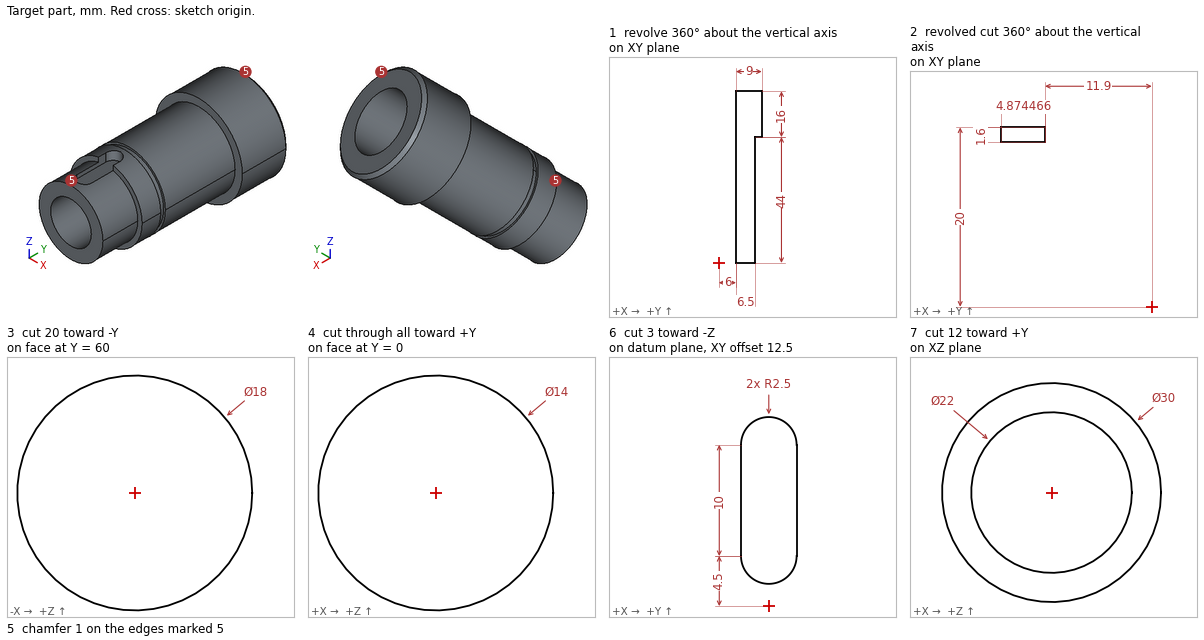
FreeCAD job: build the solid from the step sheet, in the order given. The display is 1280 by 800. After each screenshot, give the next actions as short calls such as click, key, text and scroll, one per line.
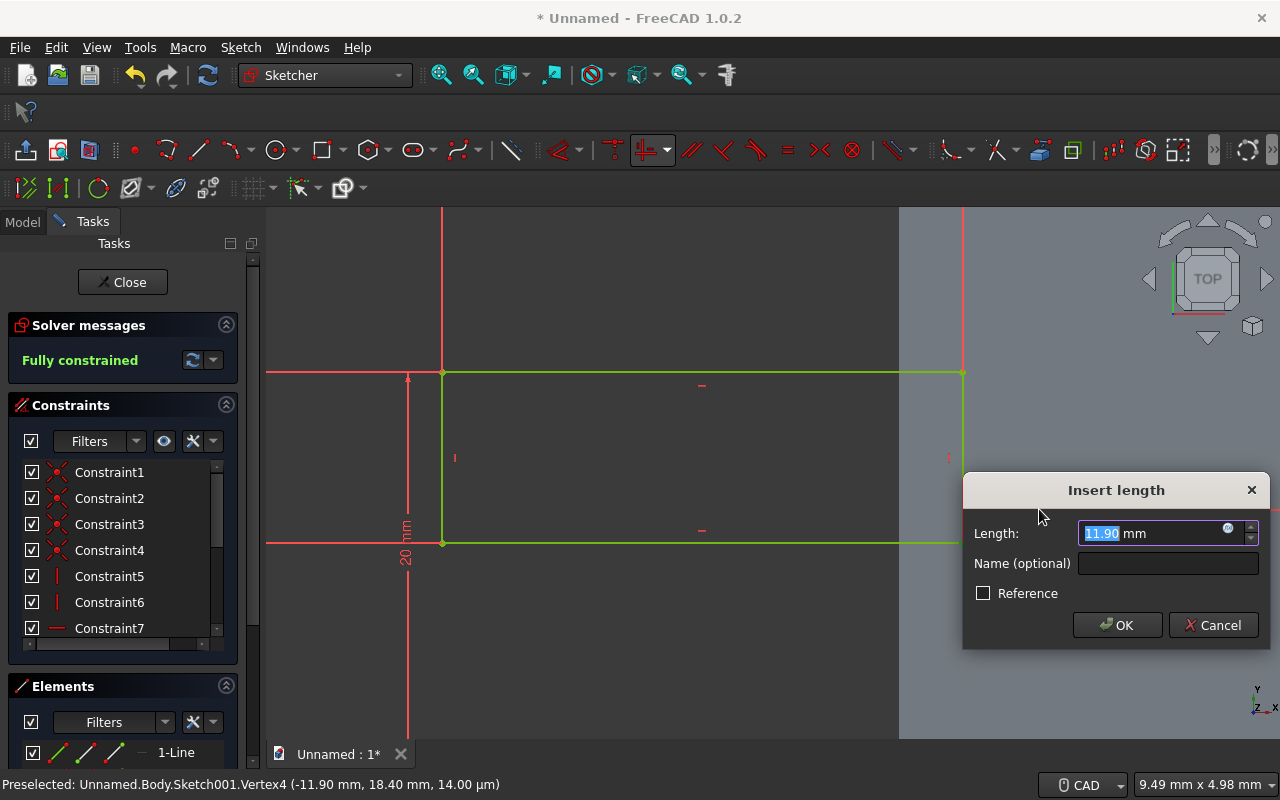
text(11.9)
key(Return)
key(Escape)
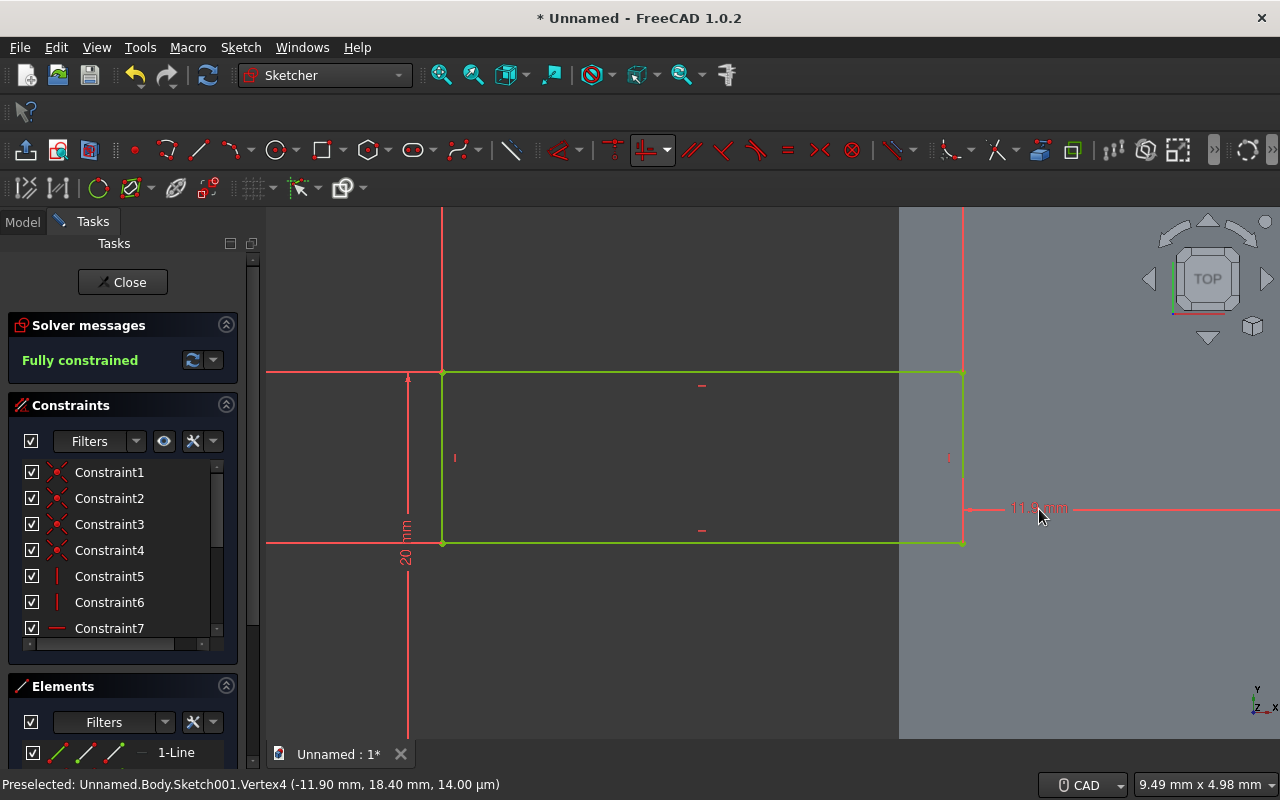
click(123, 282)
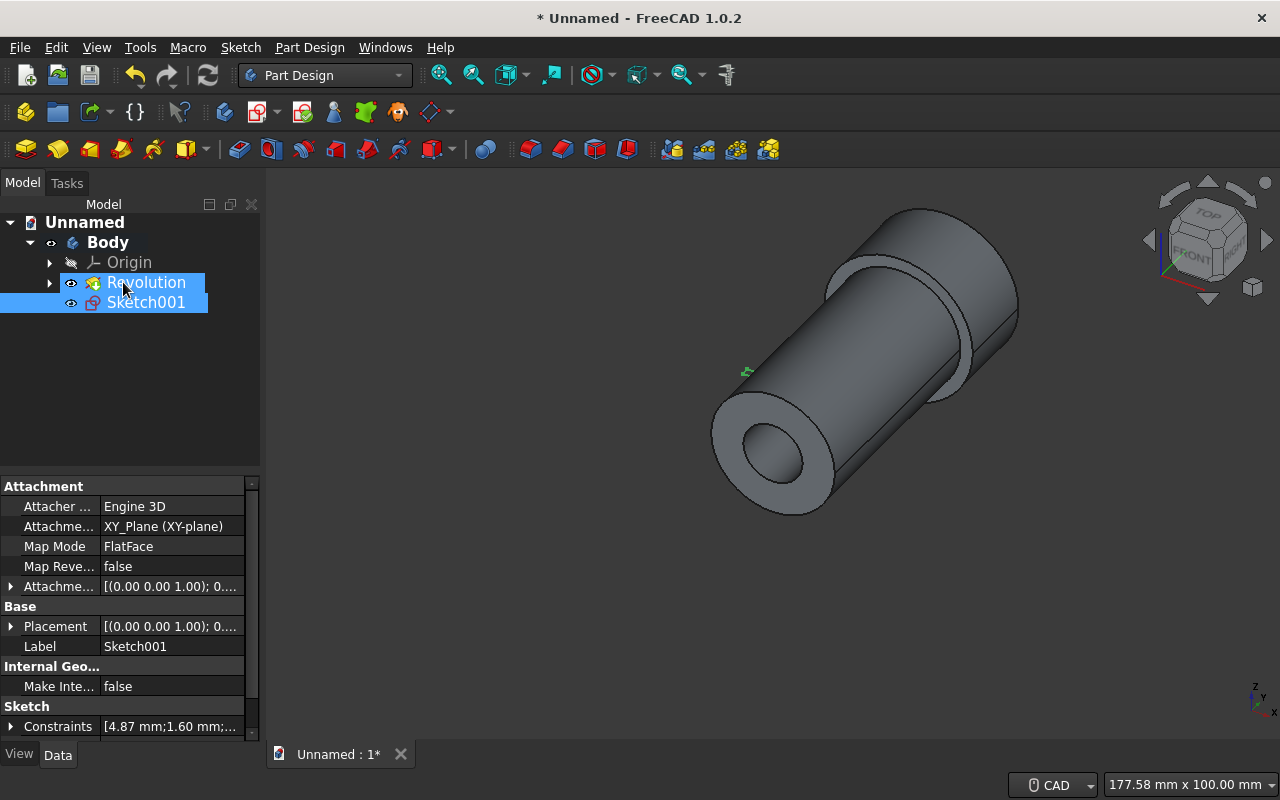
click(304, 150)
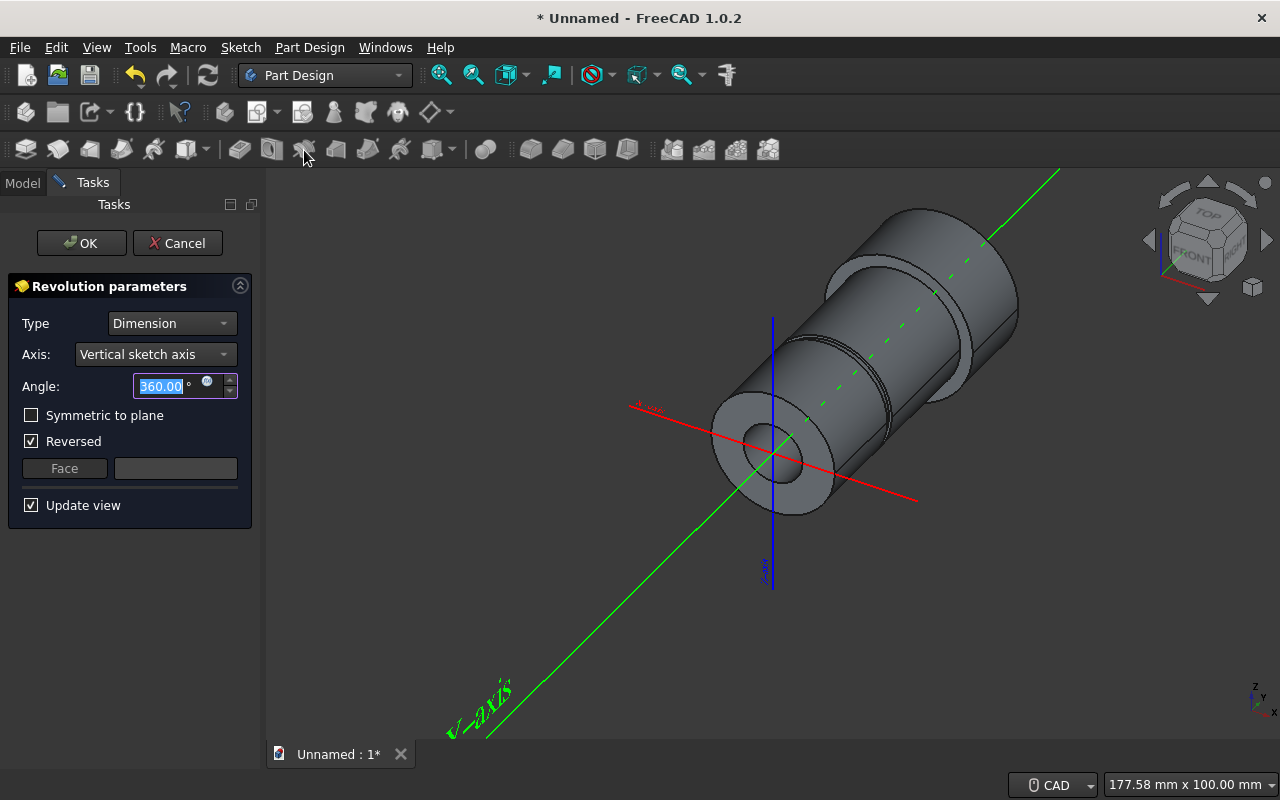
click(82, 243)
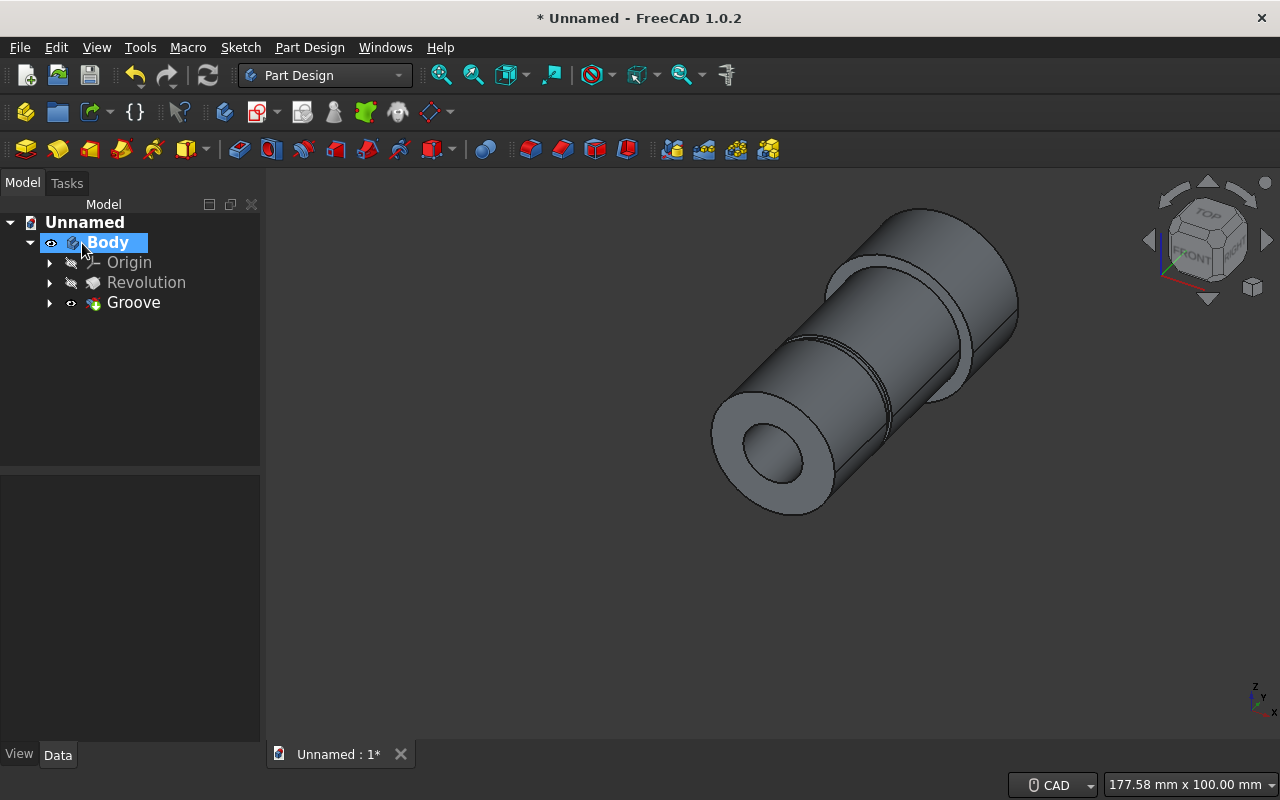
key(4)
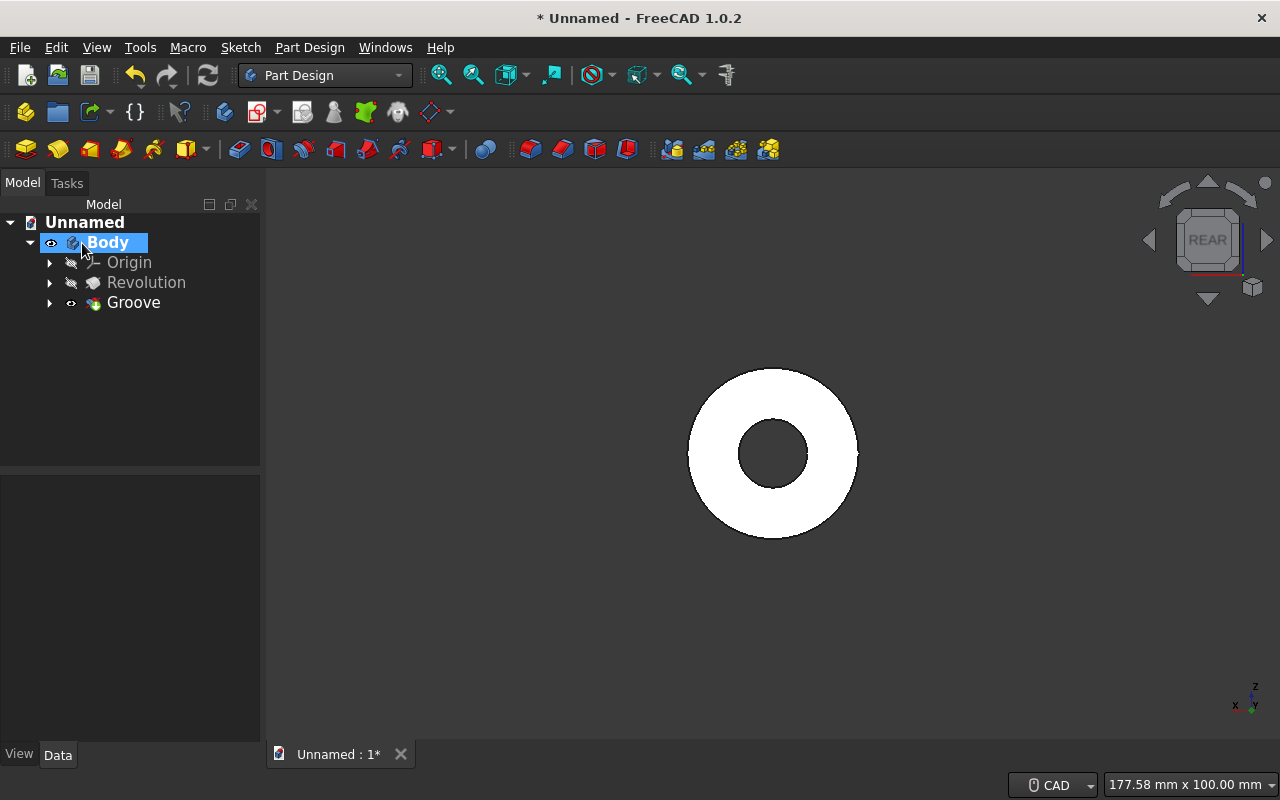
click(442, 76)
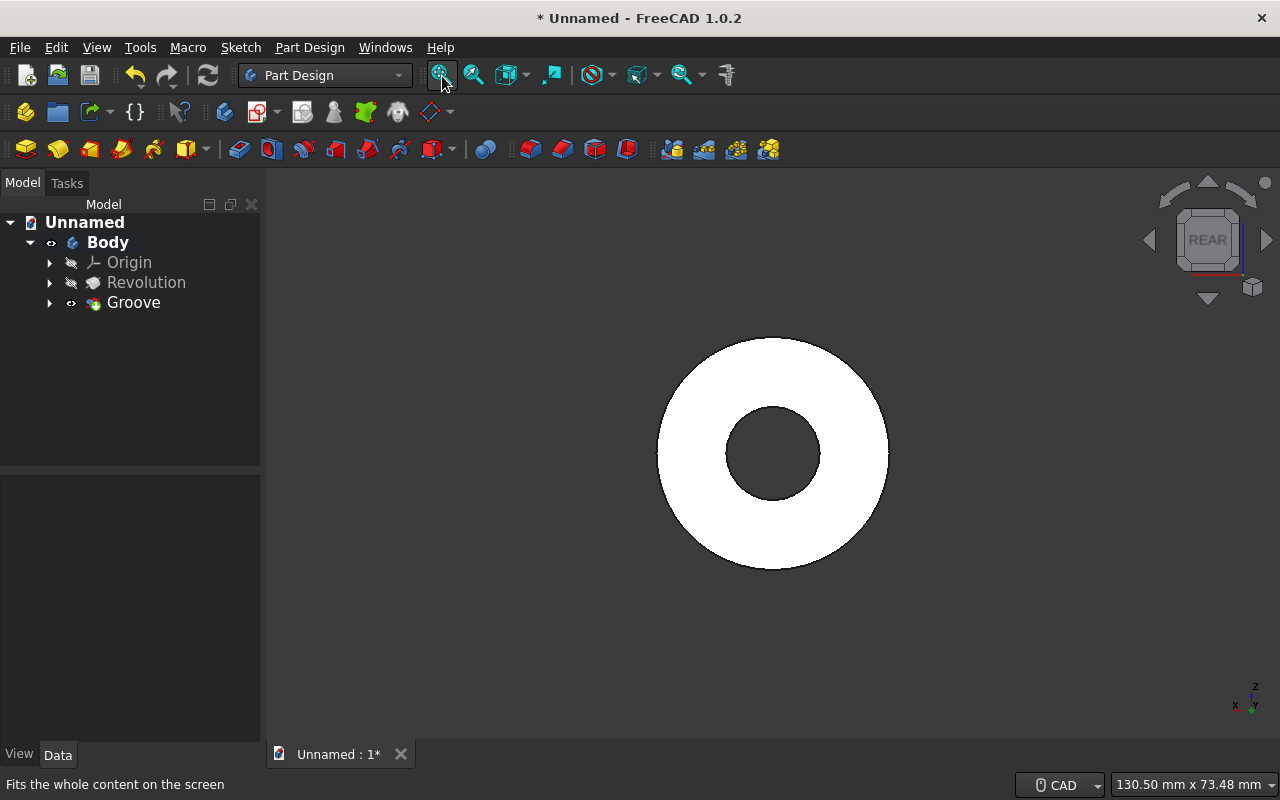
click(706, 486)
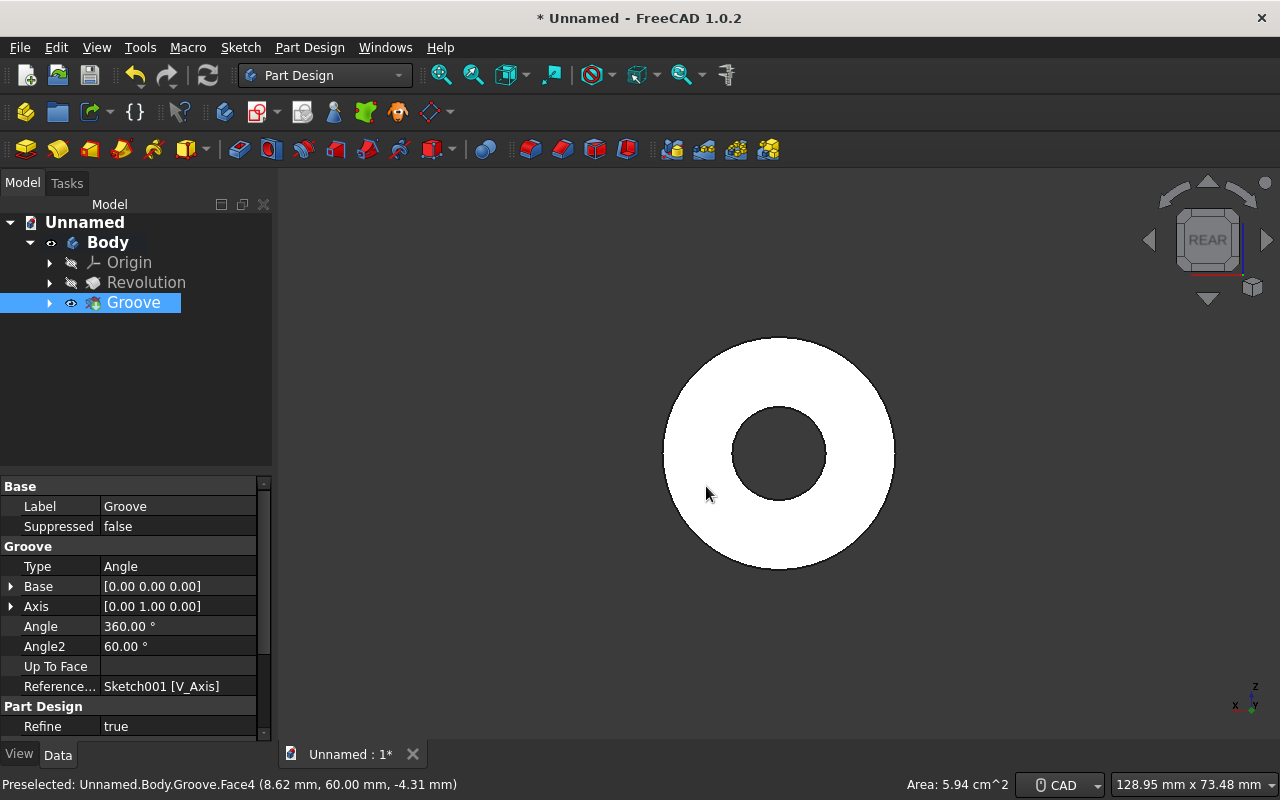
click(258, 112)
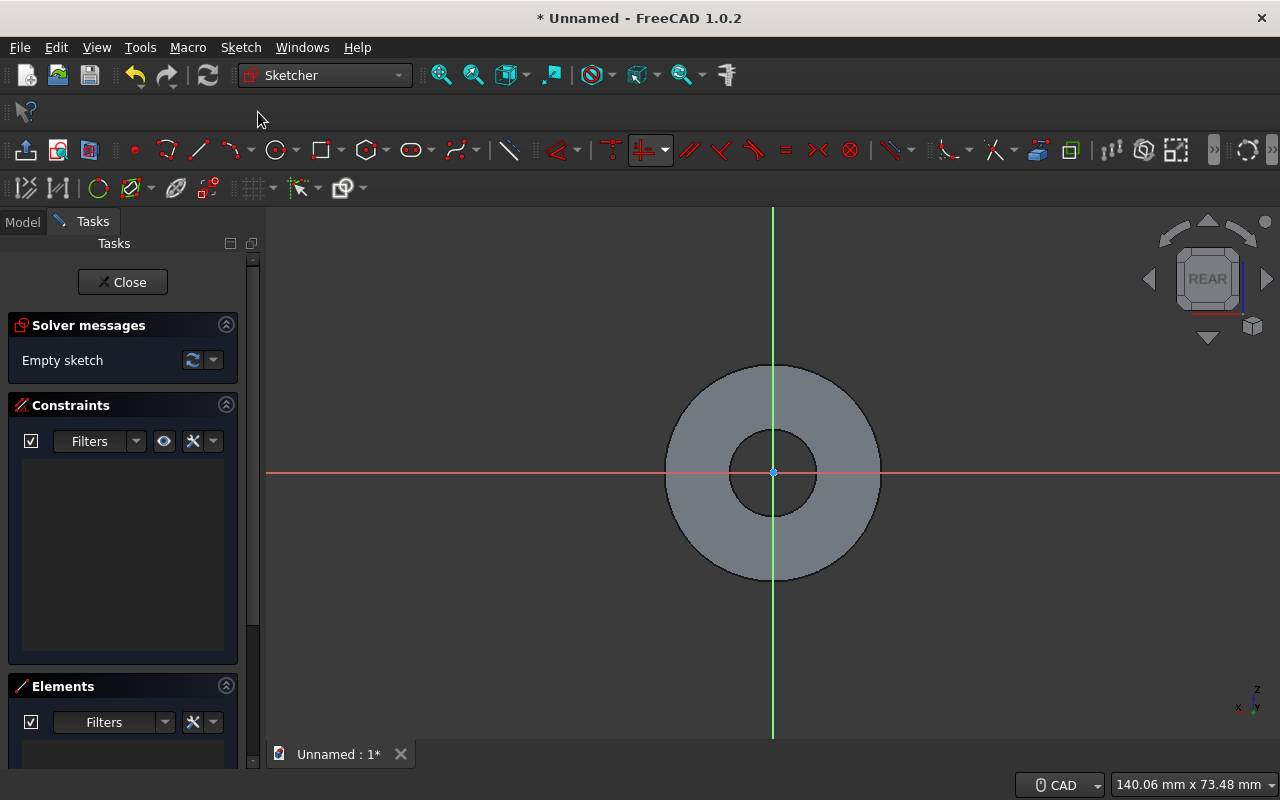
scroll(813, 473, up, 5)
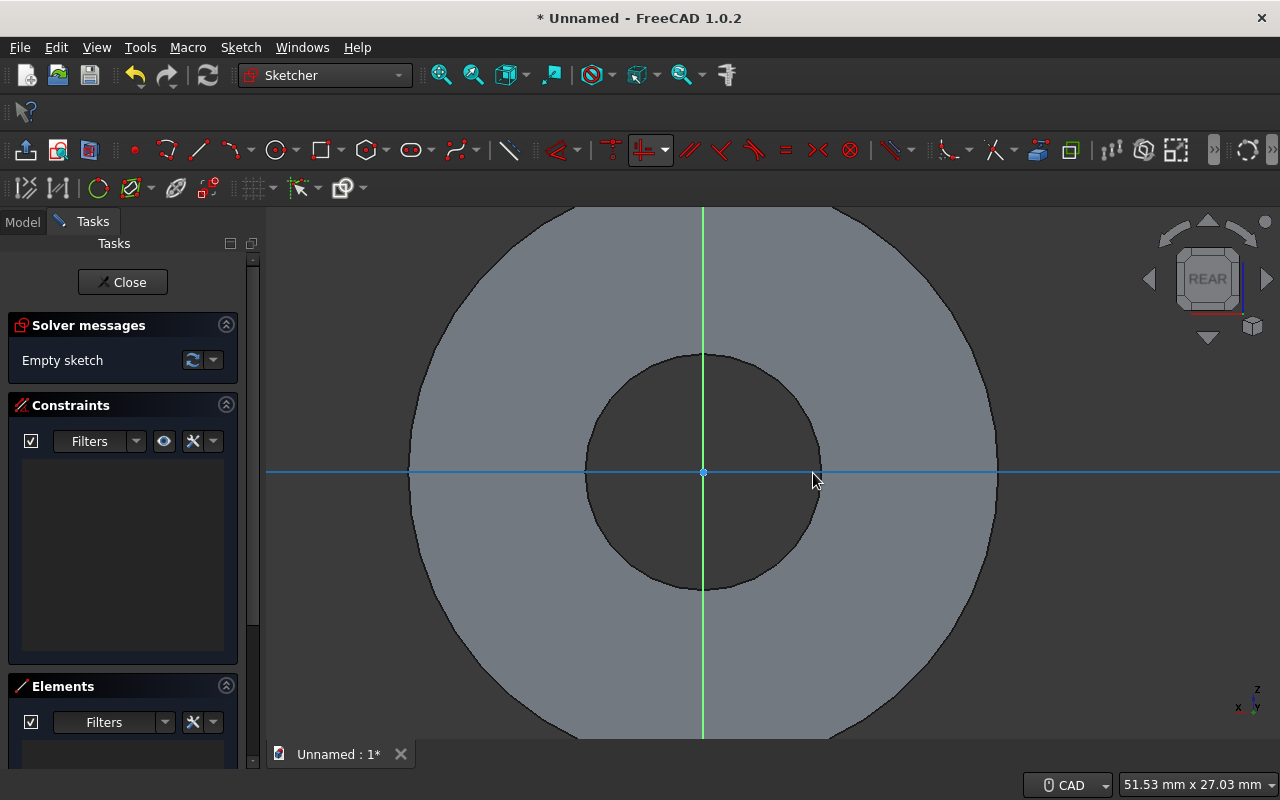
click(276, 150)